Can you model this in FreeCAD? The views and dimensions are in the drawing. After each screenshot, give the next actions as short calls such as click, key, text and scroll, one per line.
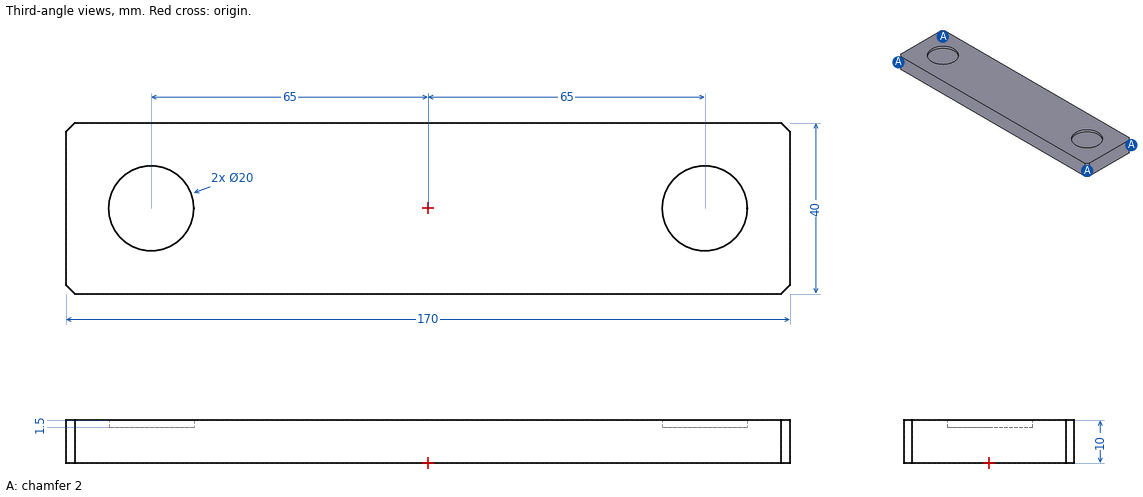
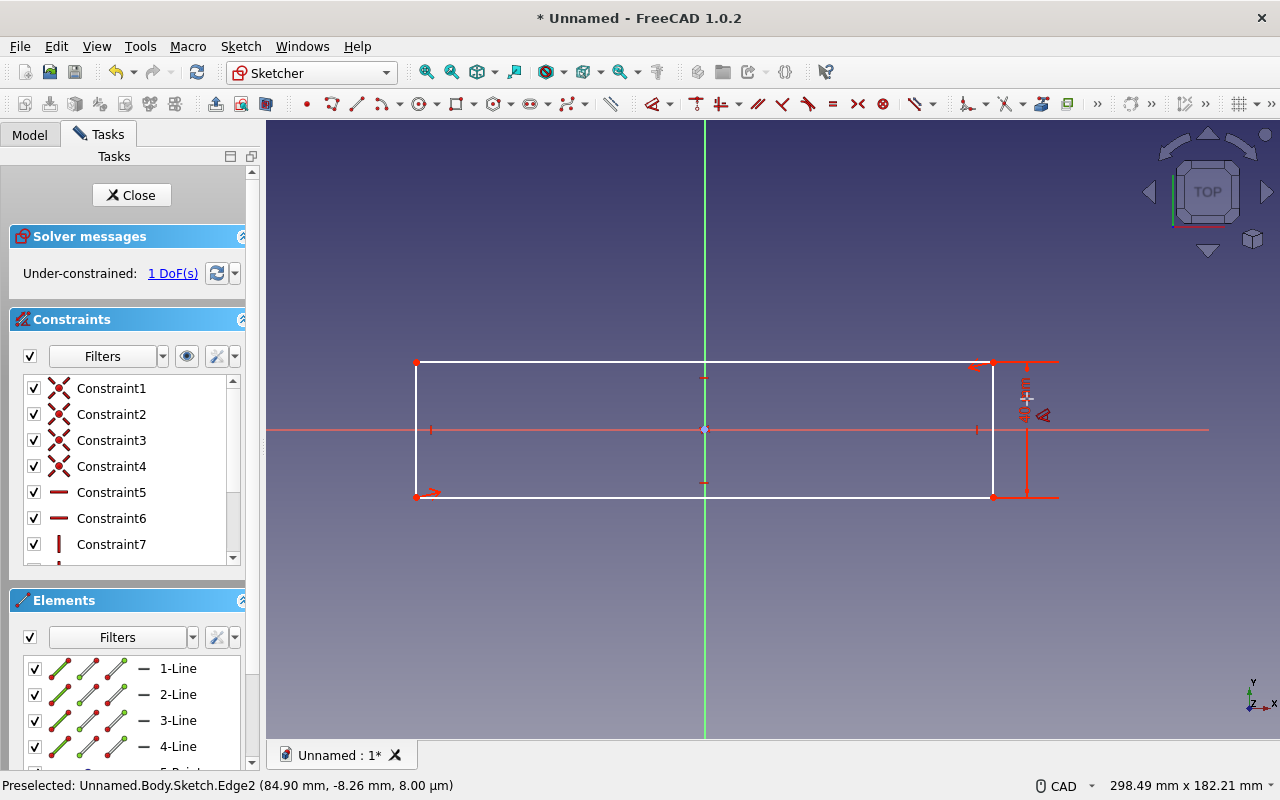
click(589, 498)
click(572, 532)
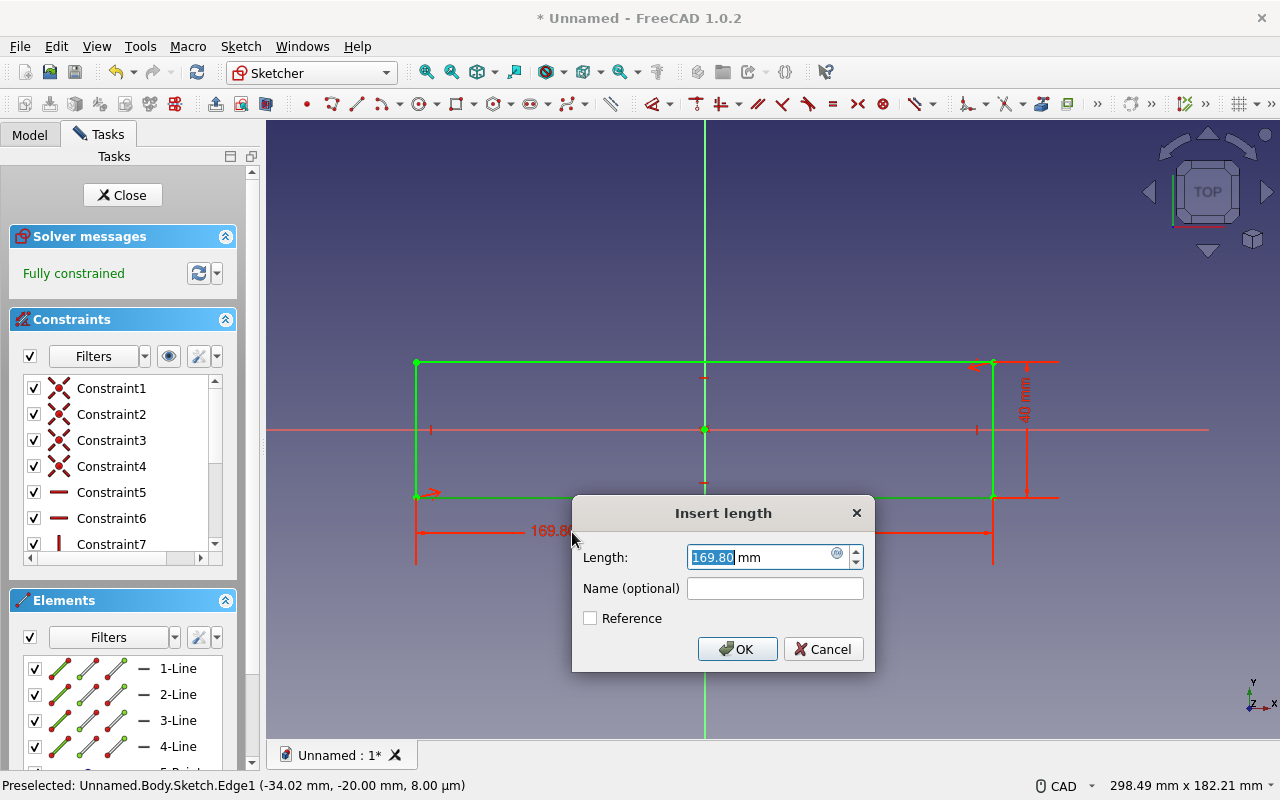
text(170)
key(Return)
key(Escape)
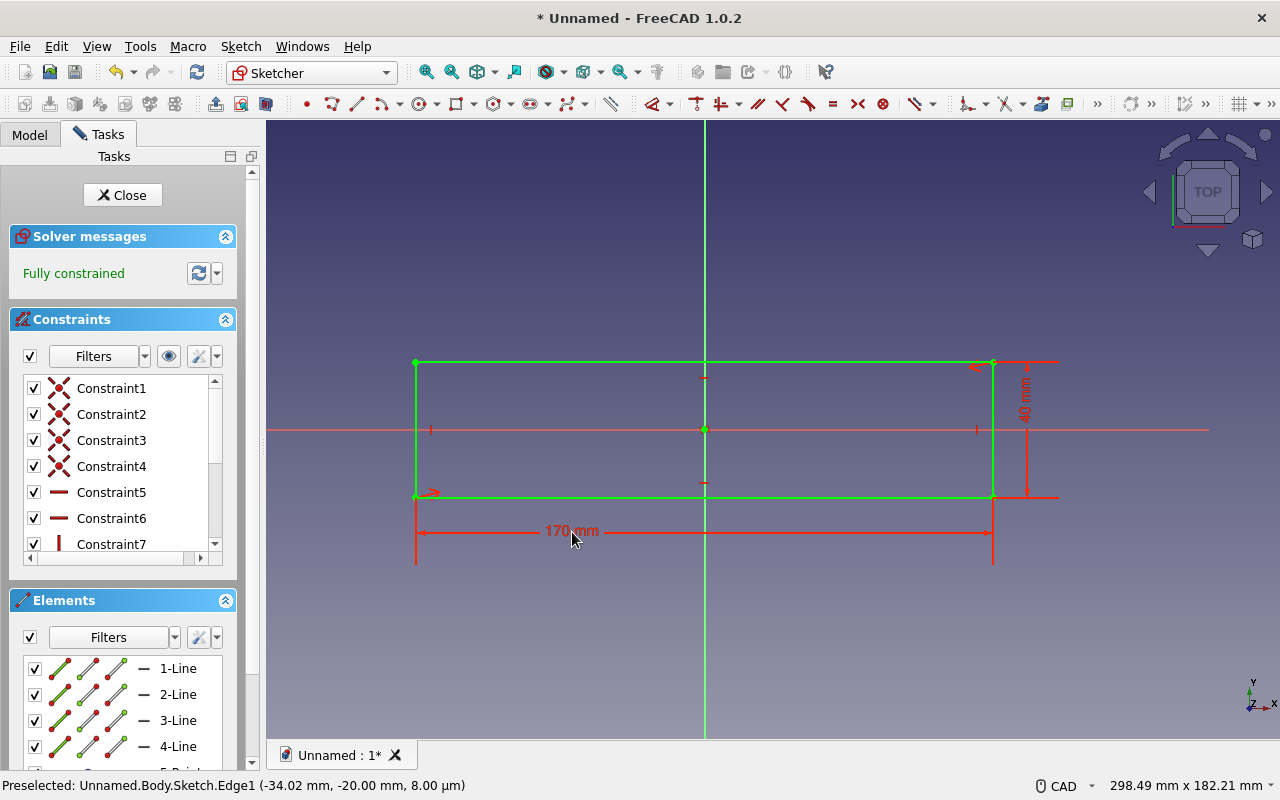
click(123, 195)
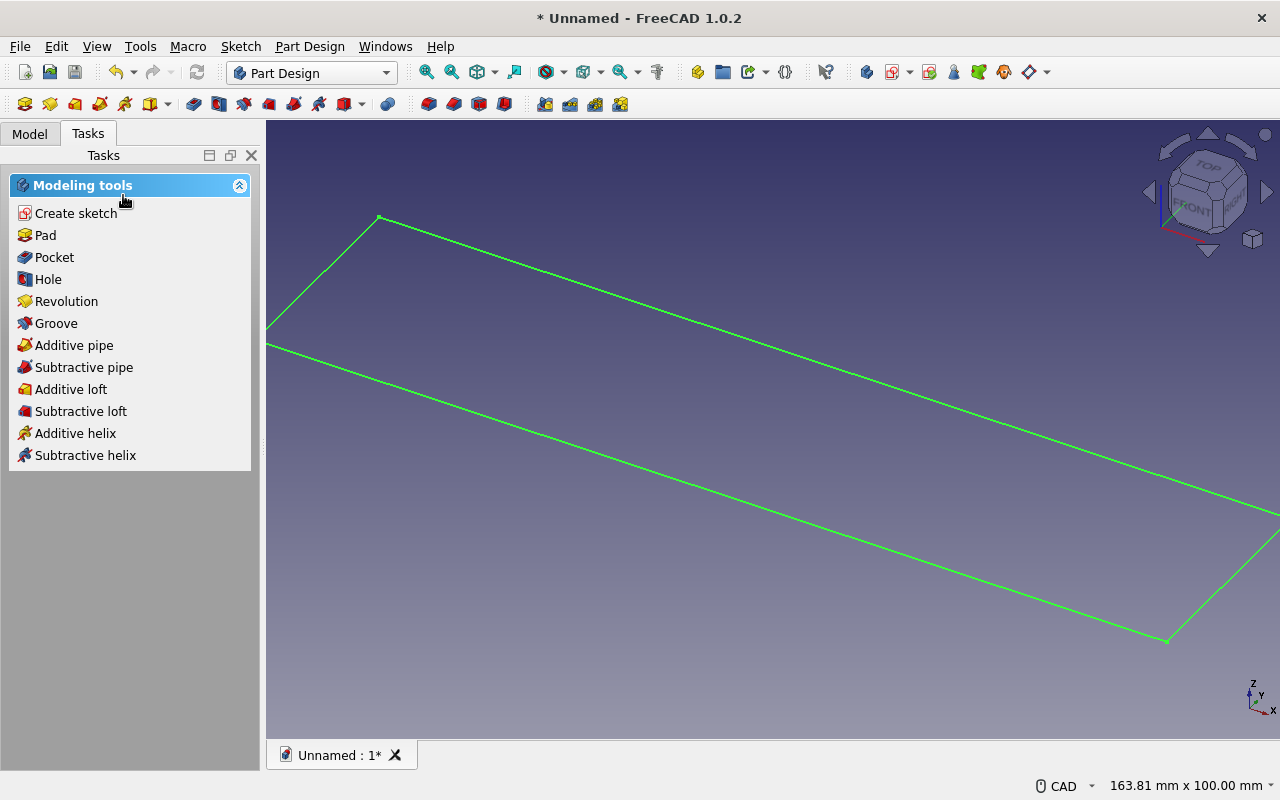
click(25, 104)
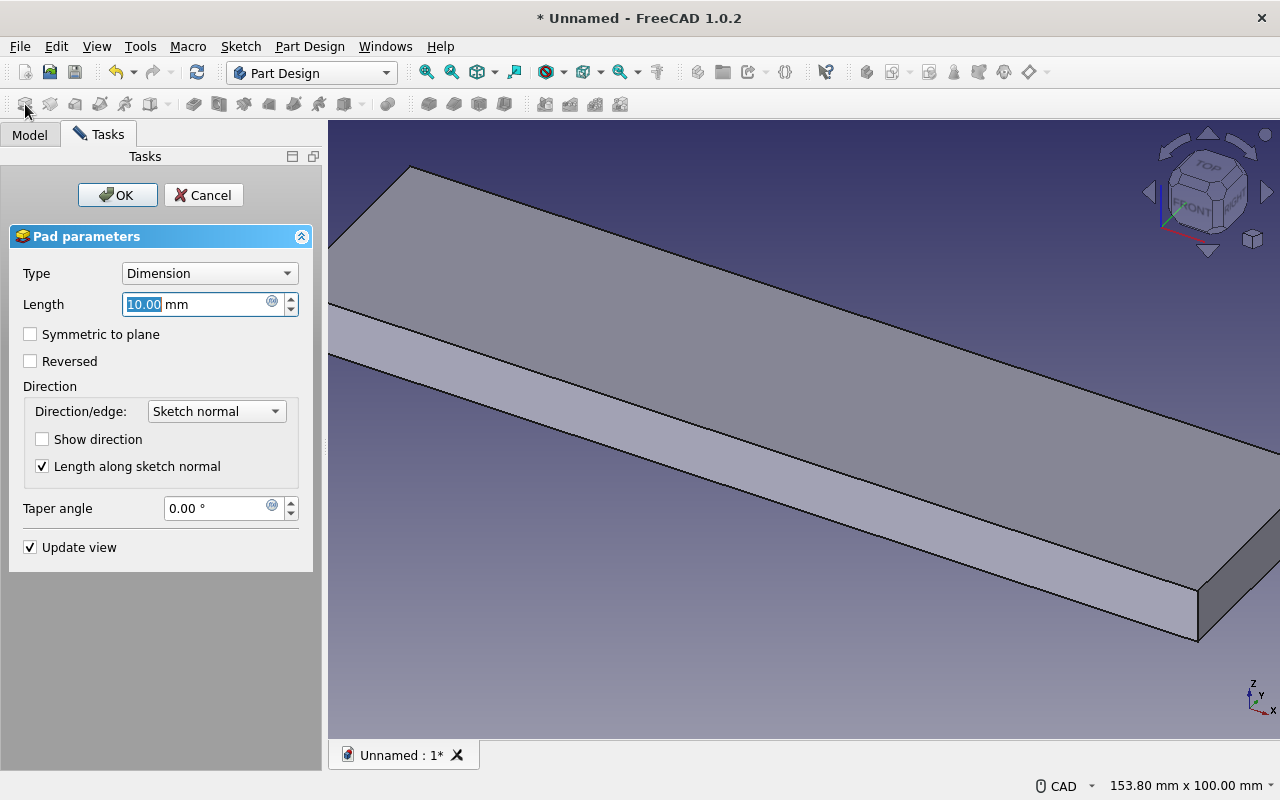
text(10)
key(Tab)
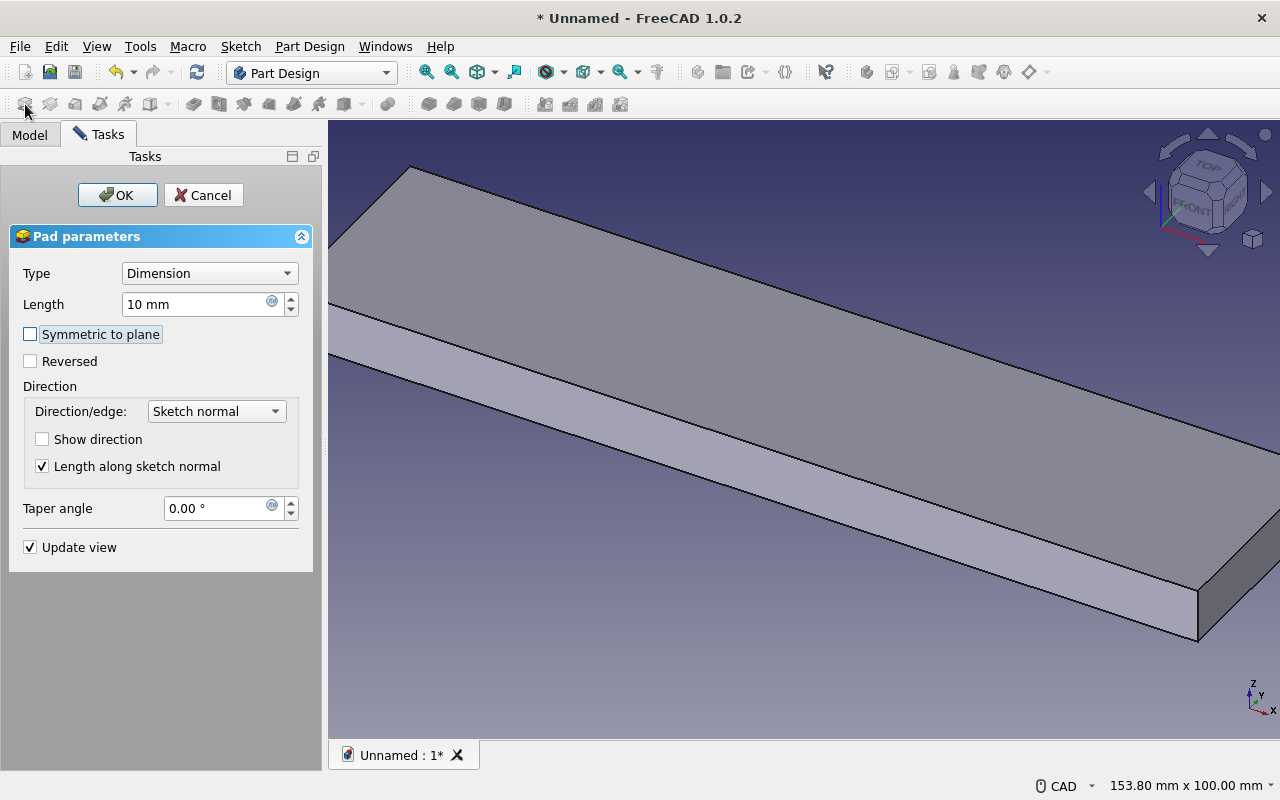
click(118, 195)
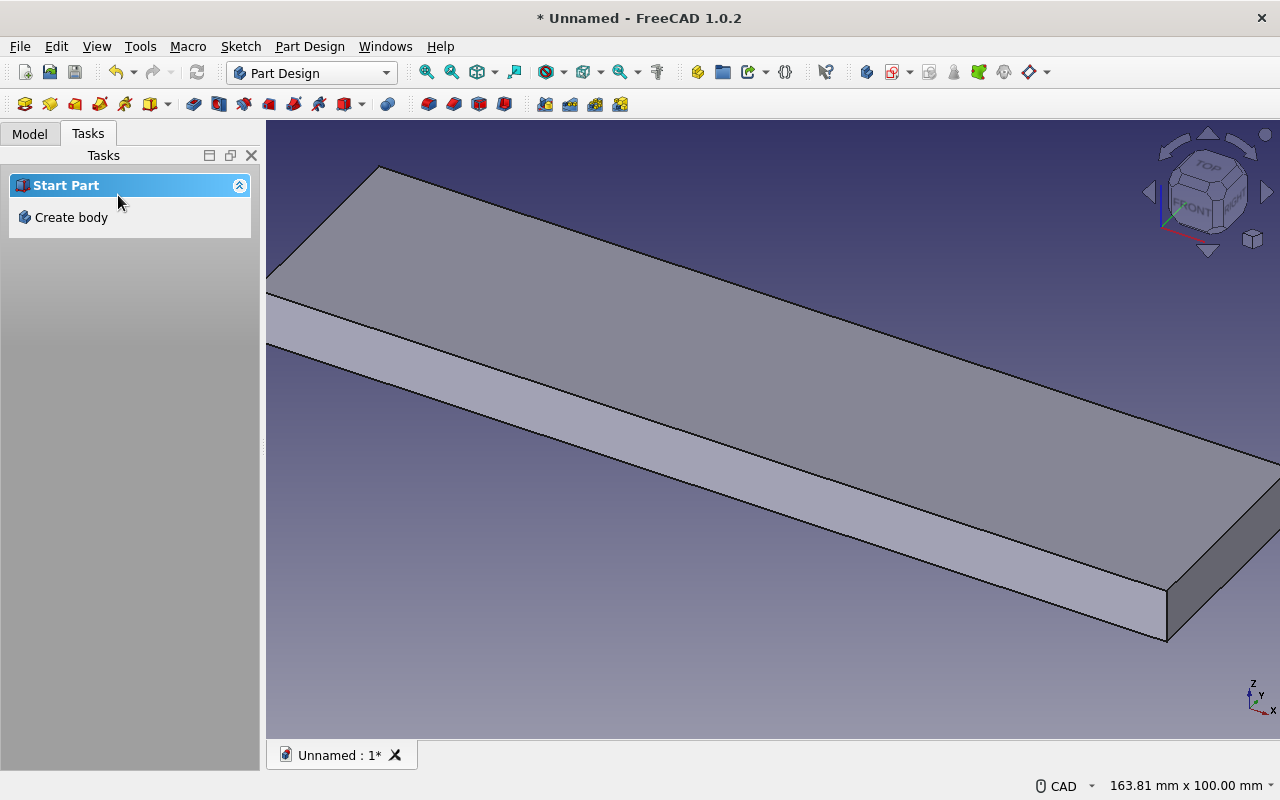
key(v)
key(f)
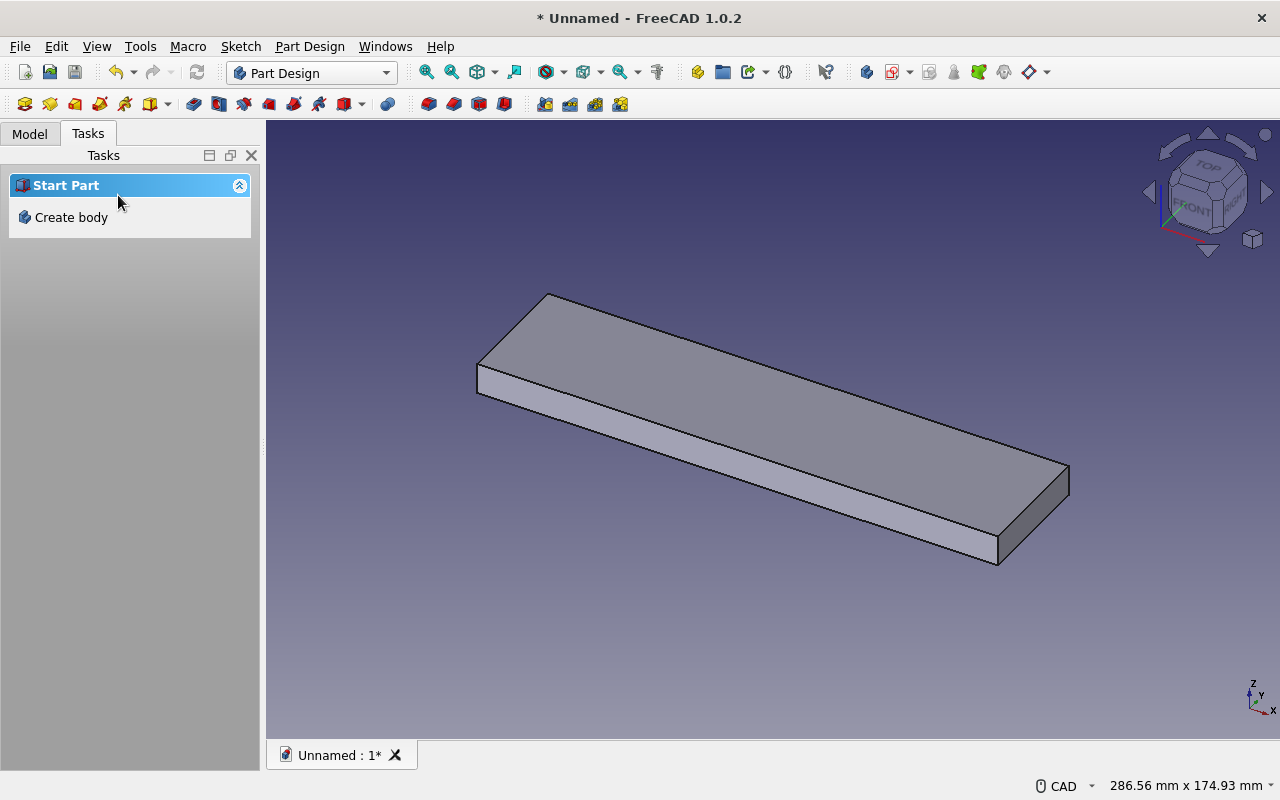
click(922, 463)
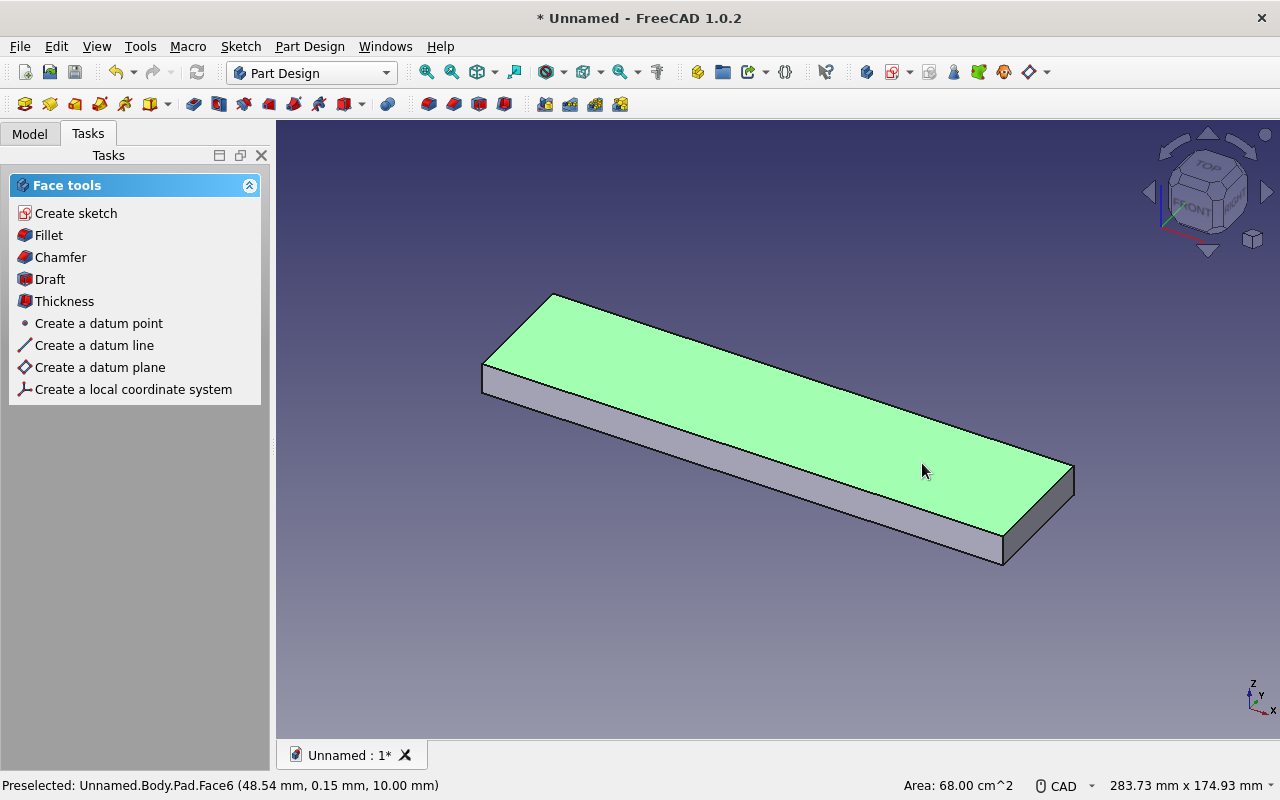
click(892, 72)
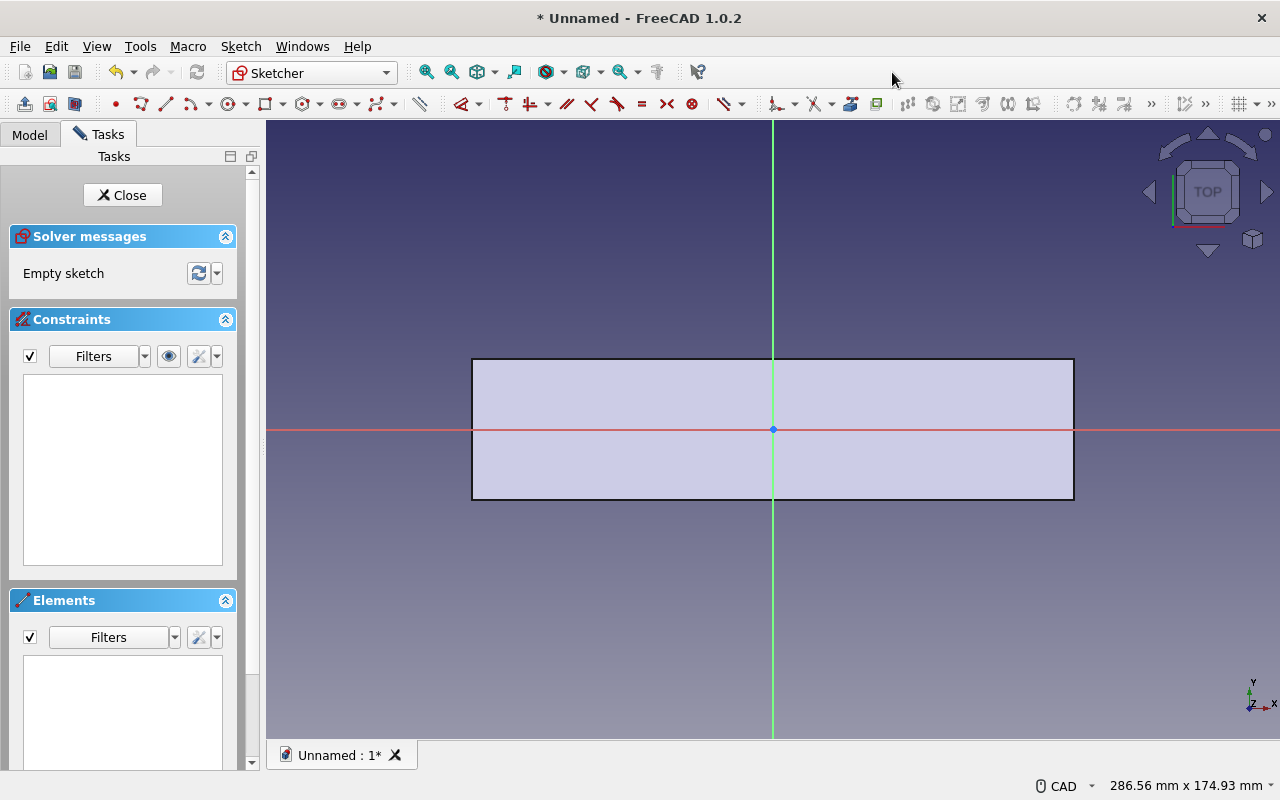
key(g)
key(c)